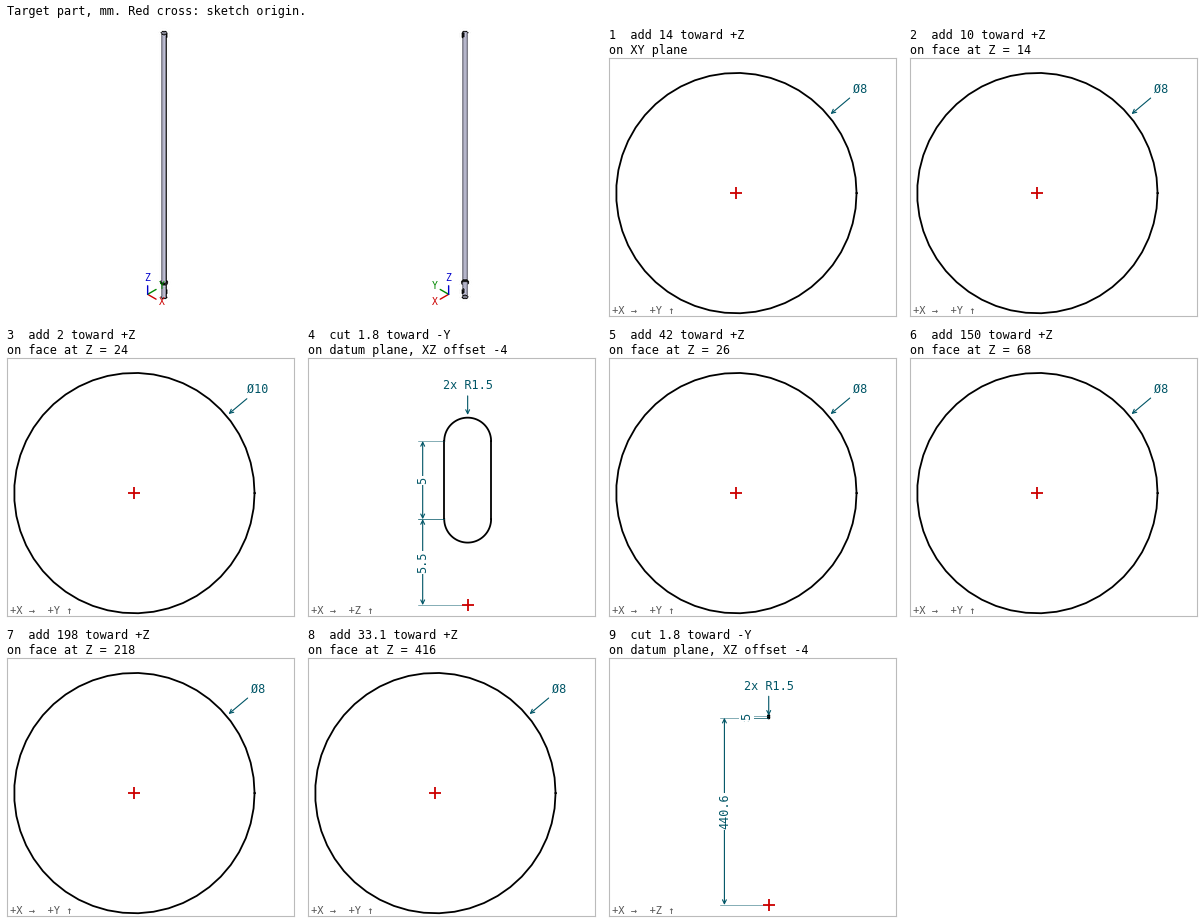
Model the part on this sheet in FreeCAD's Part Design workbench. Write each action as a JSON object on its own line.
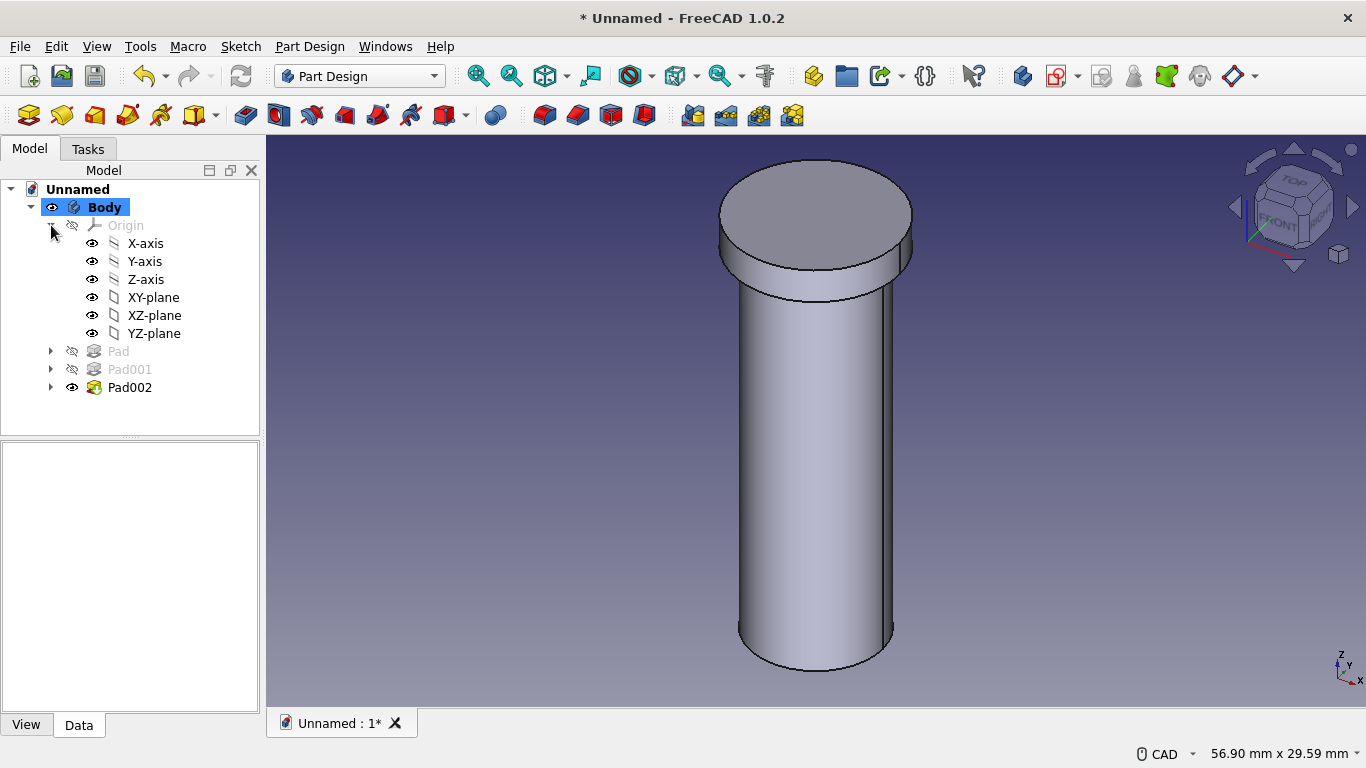
{"action": "left_click", "coordinate": [137, 315]}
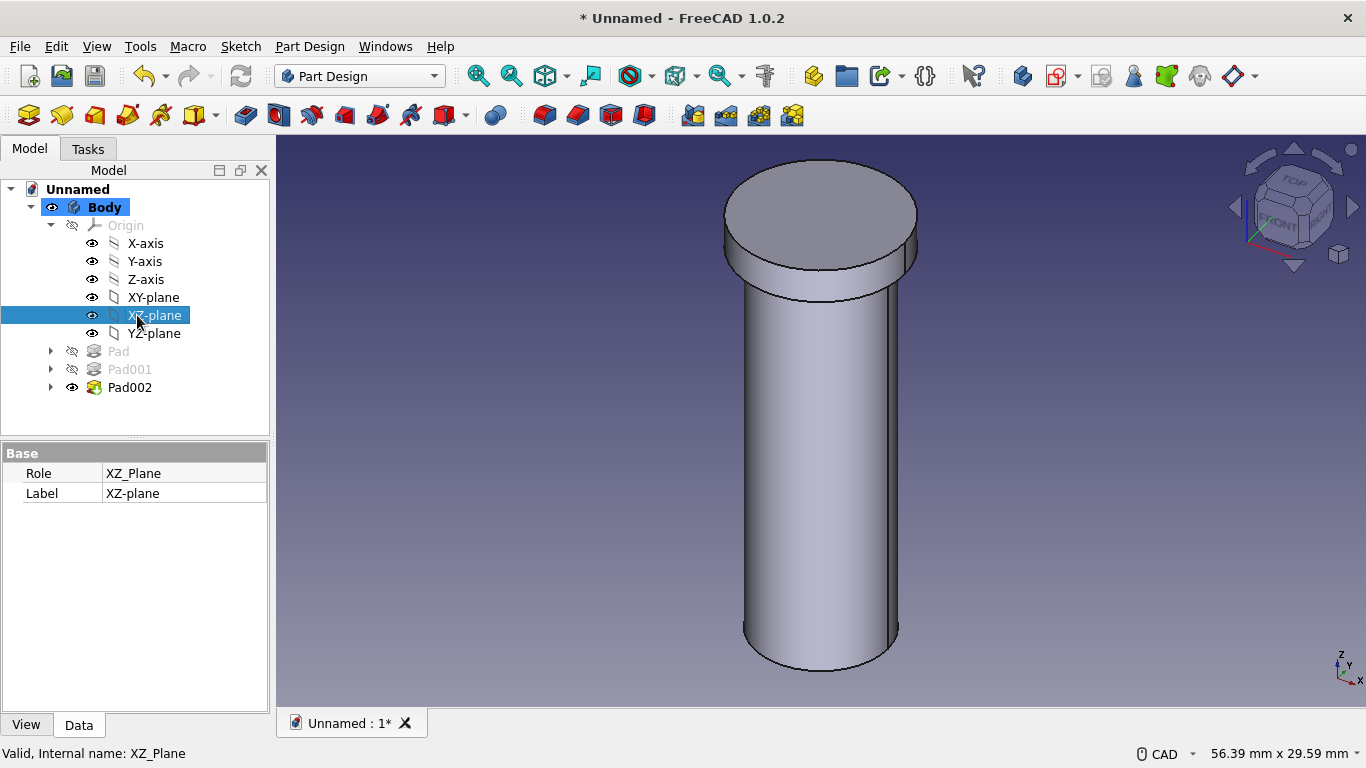
{"action": "left_click", "coordinate": [1232, 76]}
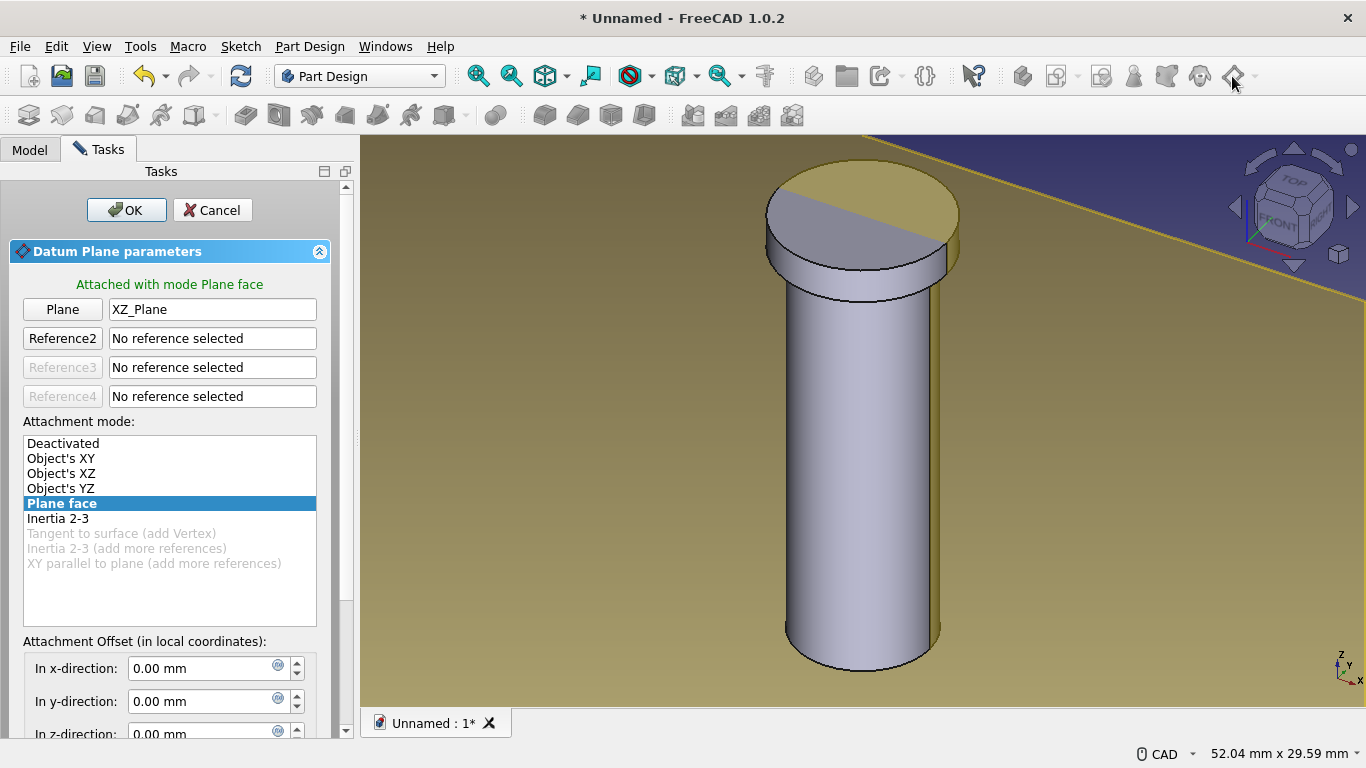
{"action": "scroll", "coordinate": [346, 460], "scroll_direction": "down", "scroll_amount": 2}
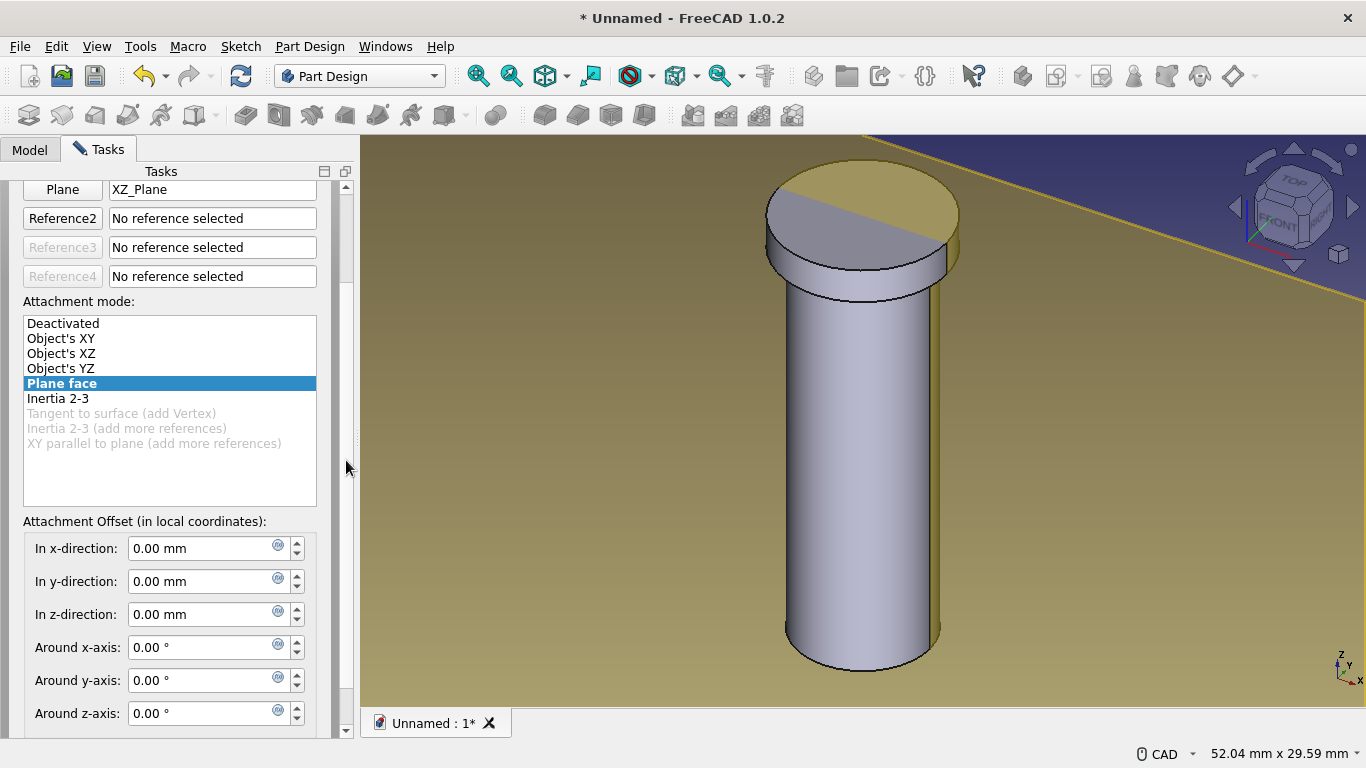
{"action": "triple_click", "coordinate": [210, 614]}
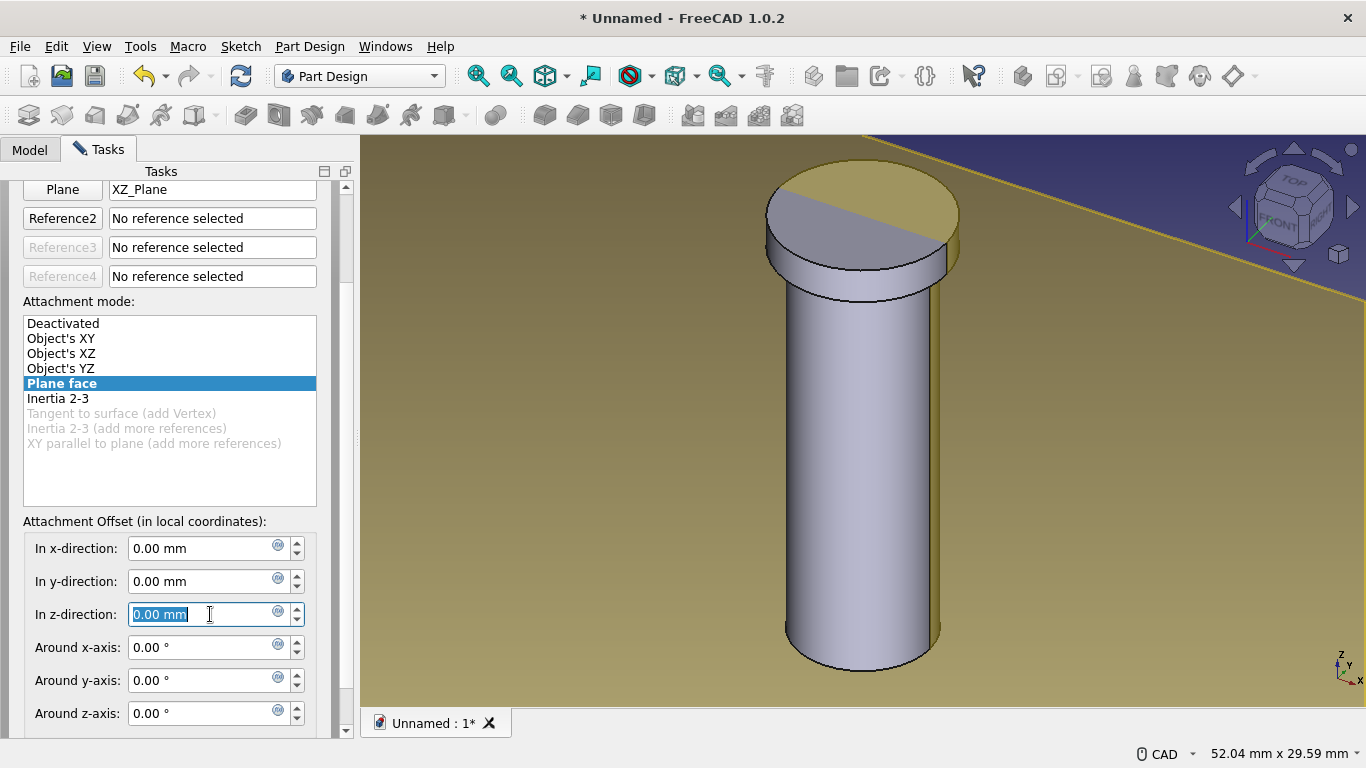
{"action": "type", "text": "-4"}
{"action": "key", "text": "Tab"}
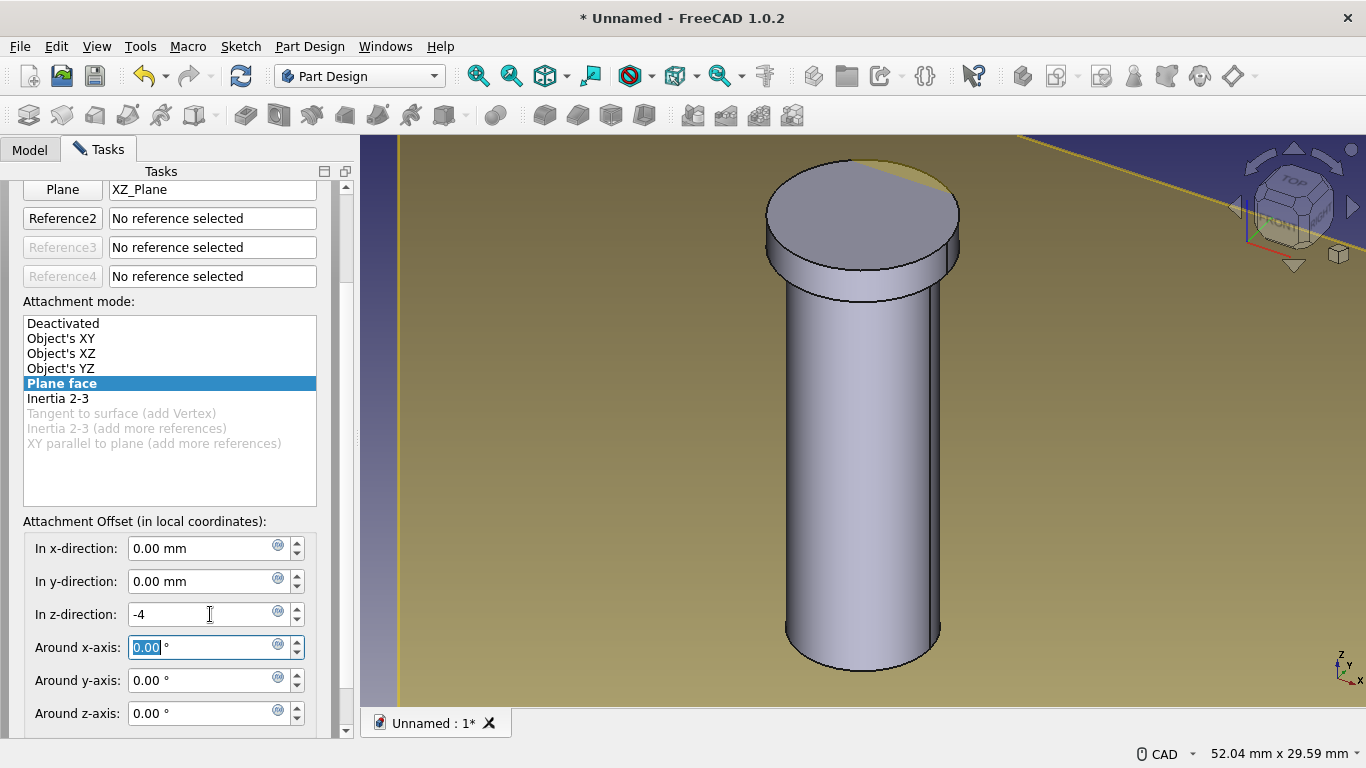
{"action": "scroll", "coordinate": [346, 460], "scroll_direction": "up", "scroll_amount": 3}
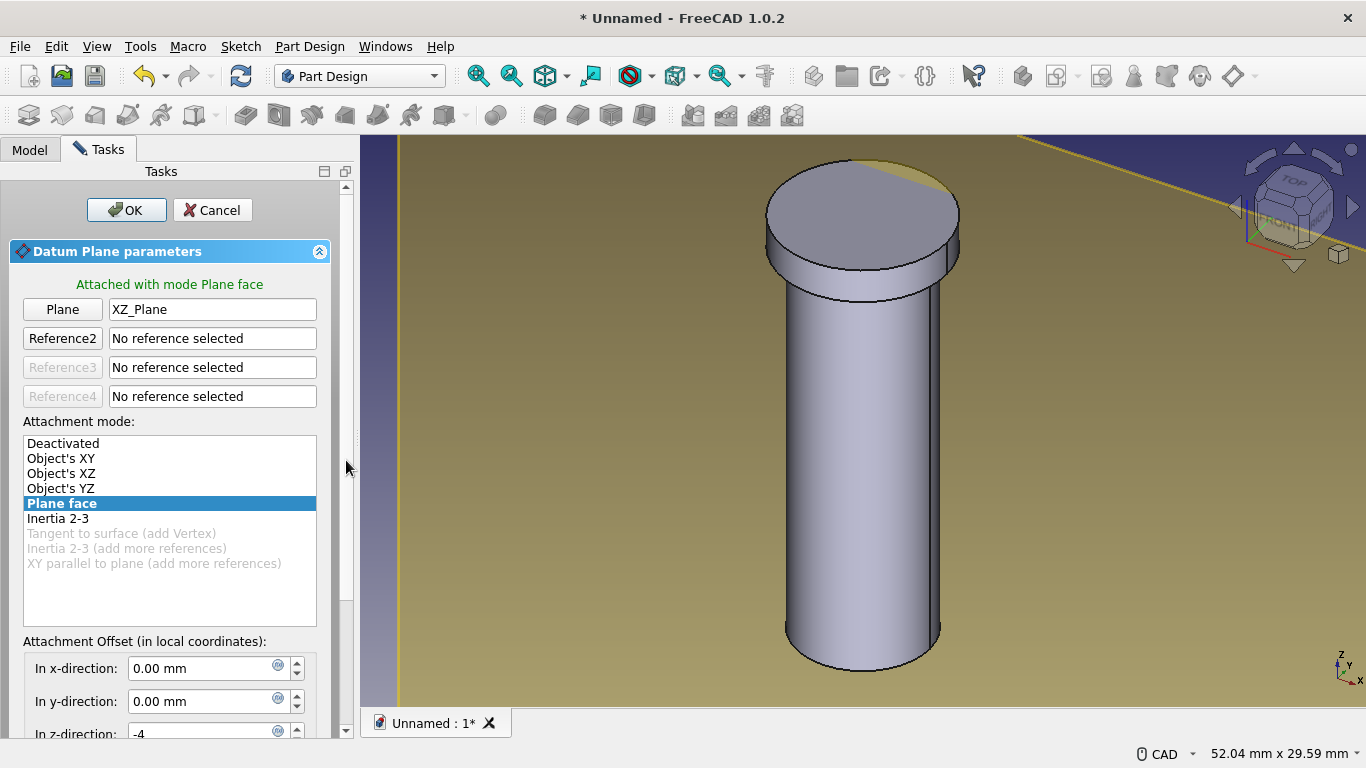
{"action": "left_click", "coordinate": [127, 210]}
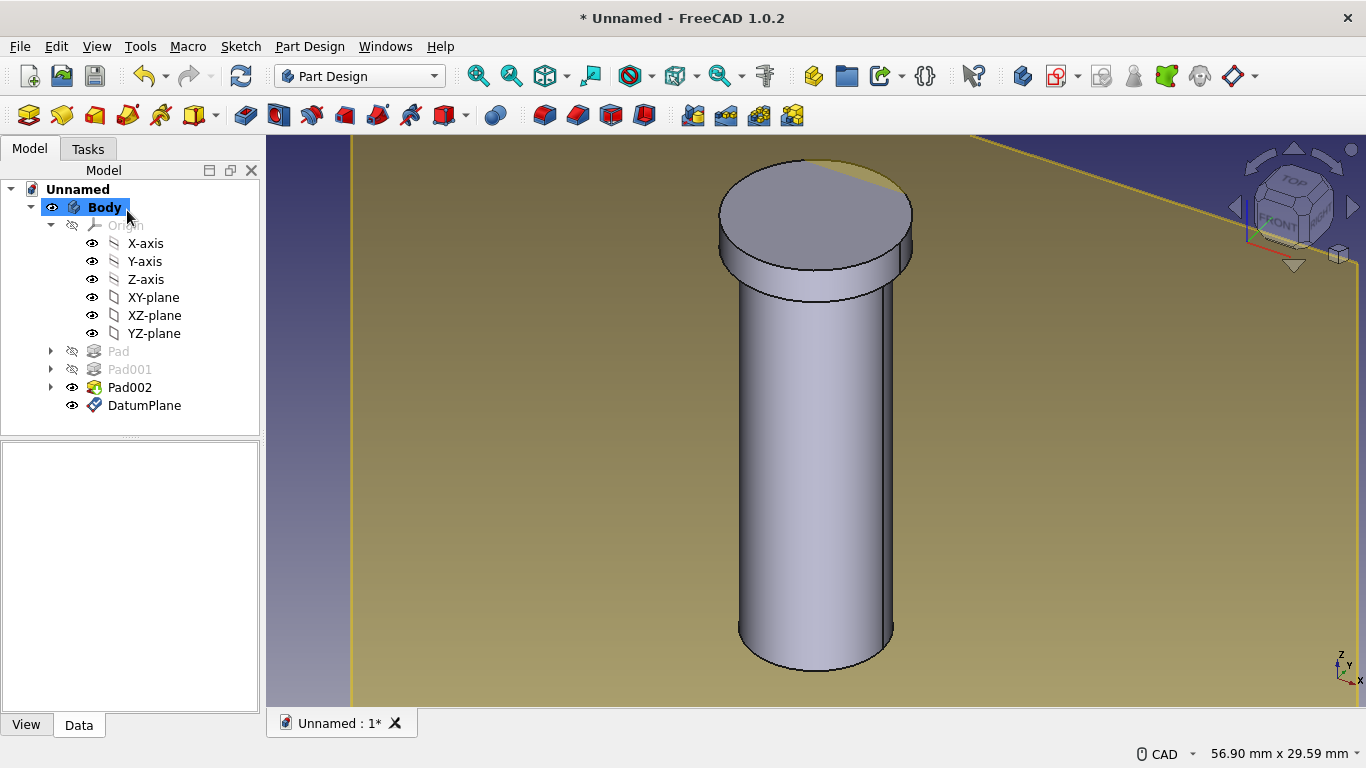
{"action": "left_click", "coordinate": [117, 405]}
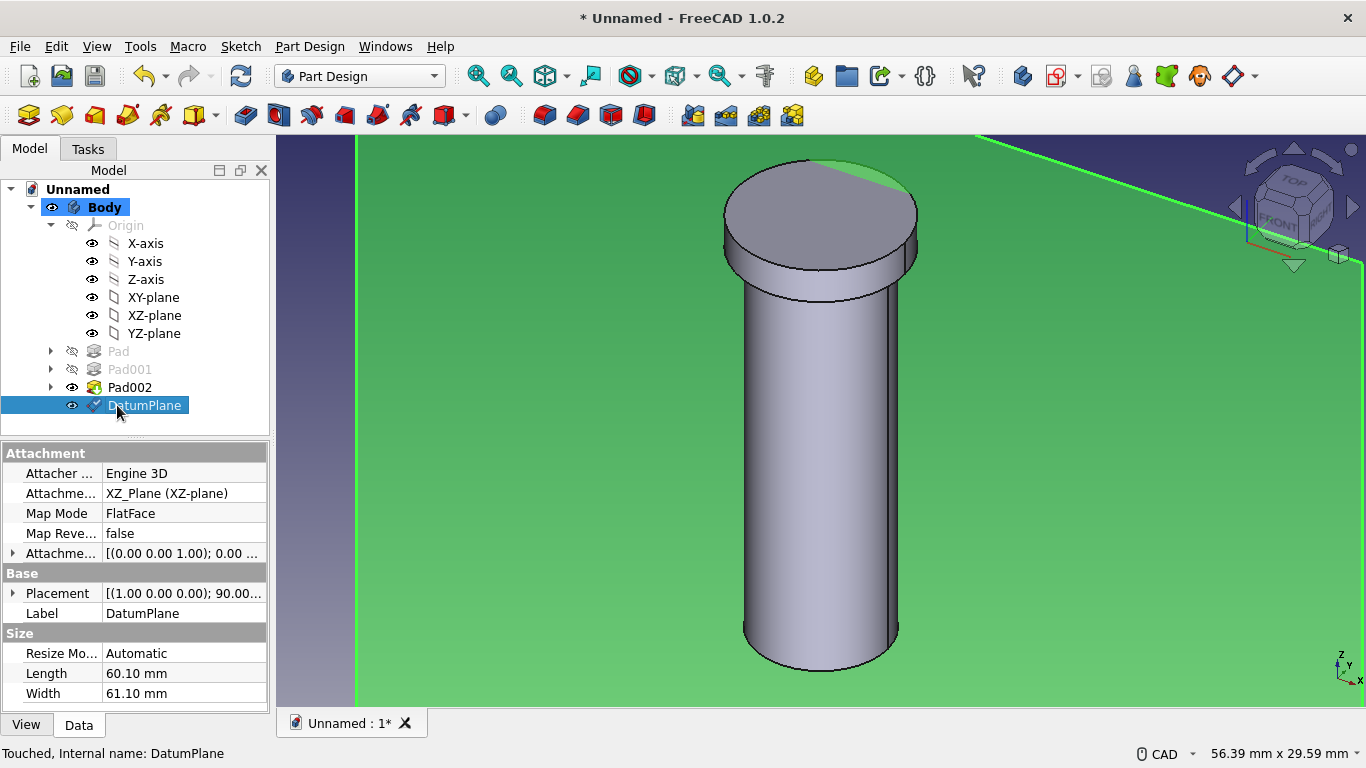
{"action": "left_click", "coordinate": [1056, 76]}